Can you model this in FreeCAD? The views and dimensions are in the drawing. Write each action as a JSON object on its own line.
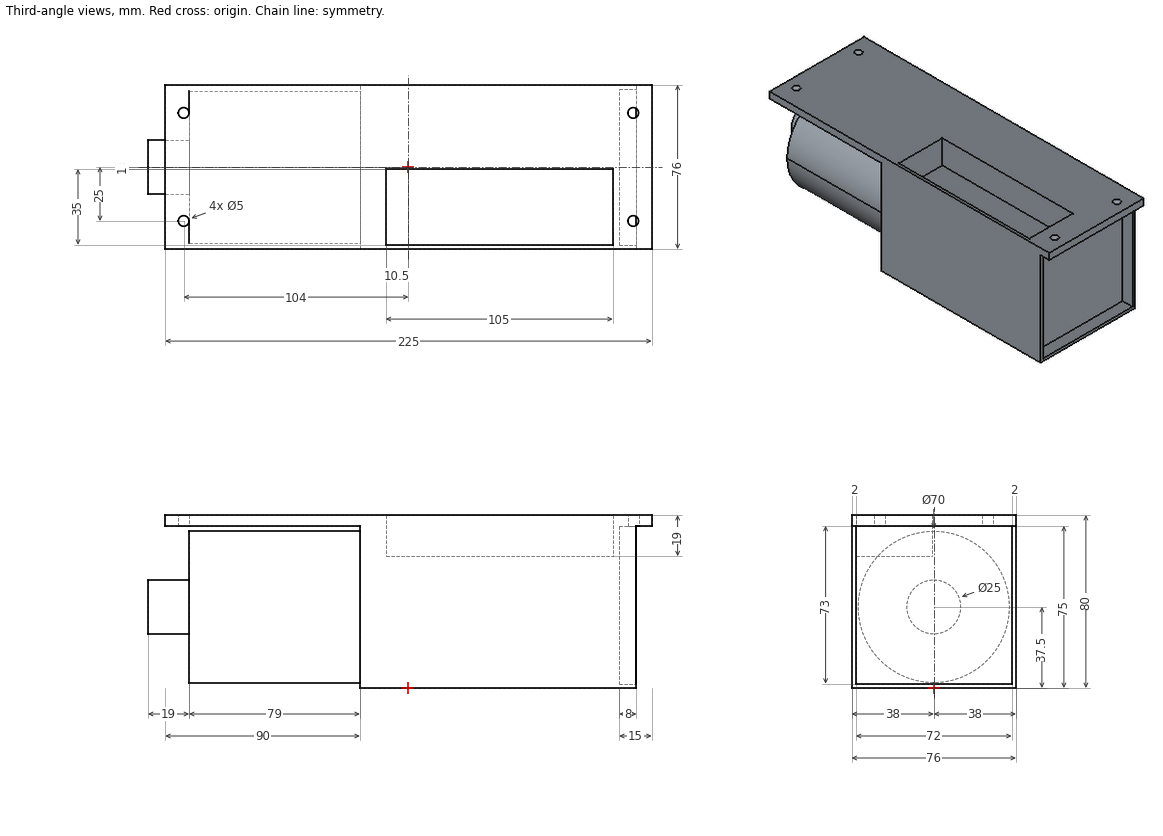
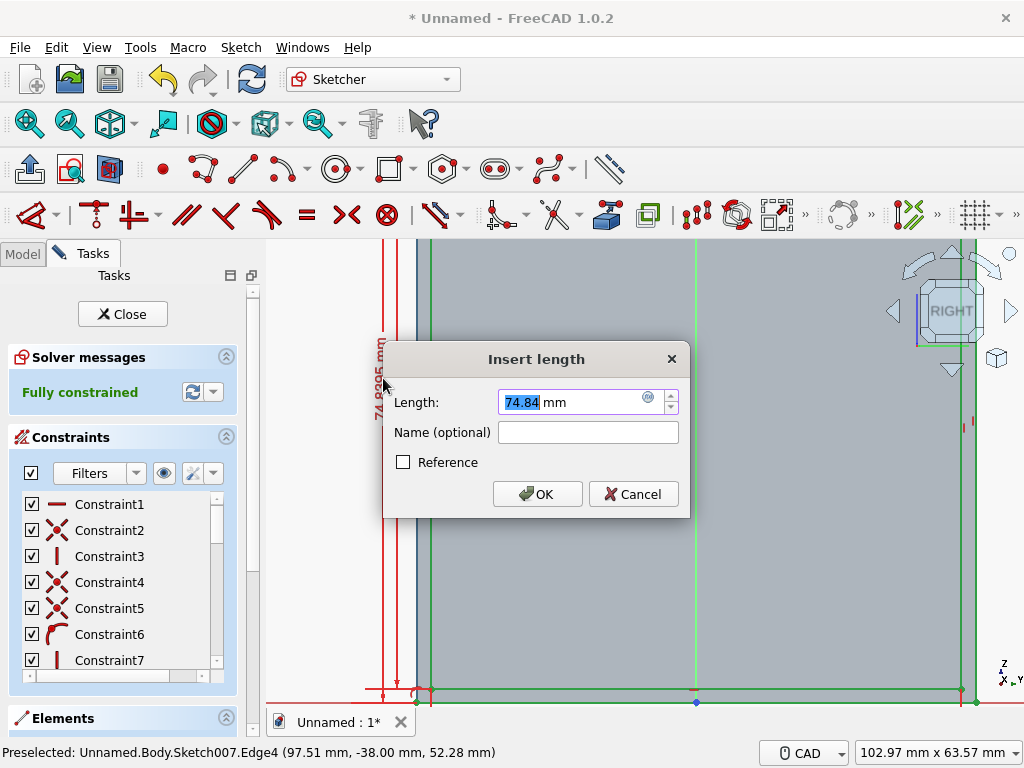
{"action": "type", "text": "75"}
{"action": "key", "text": "Return"}
{"action": "key", "text": "Escape"}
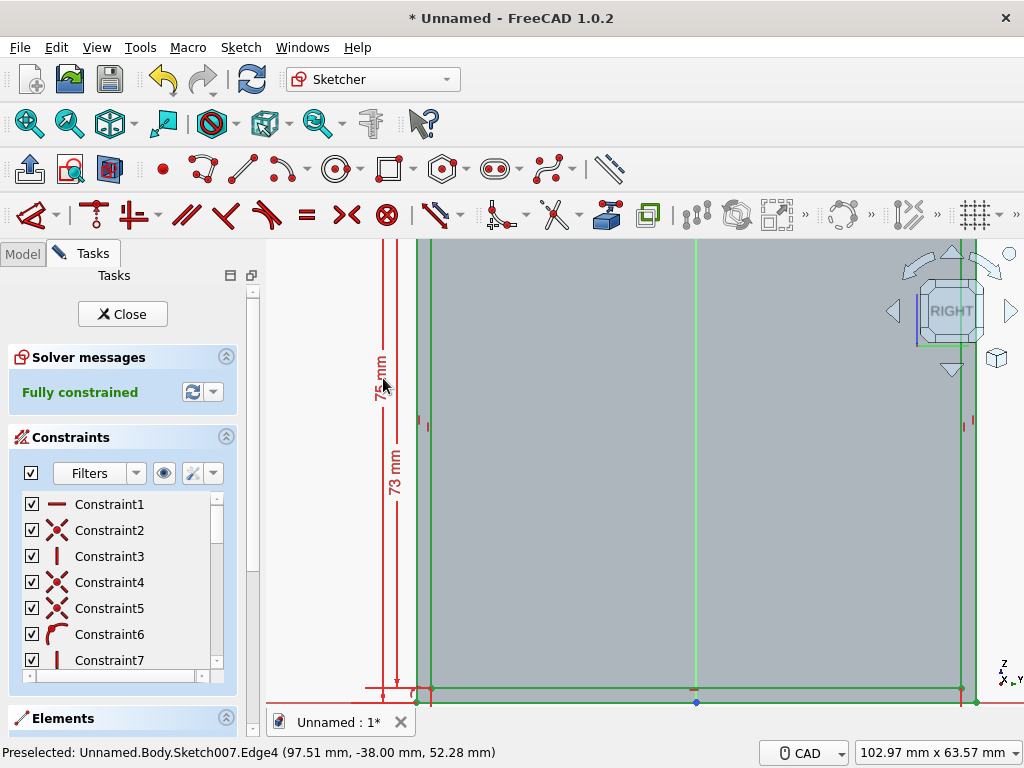
{"action": "left_click", "coordinate": [123, 314]}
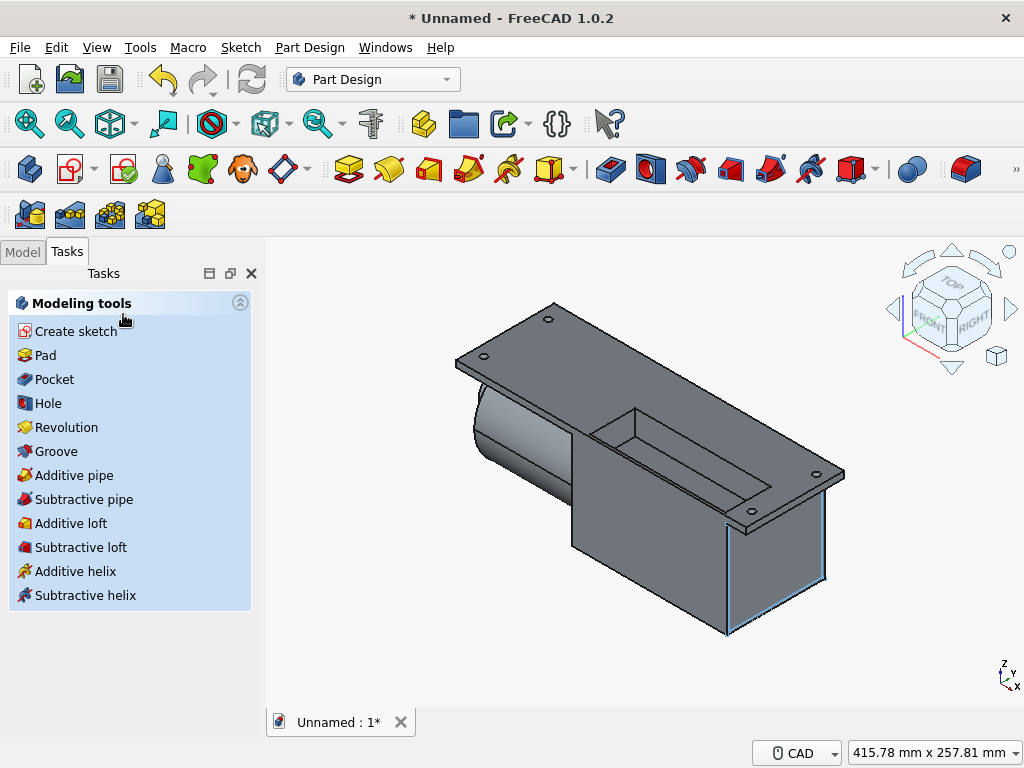
{"action": "left_click", "coordinate": [350, 170]}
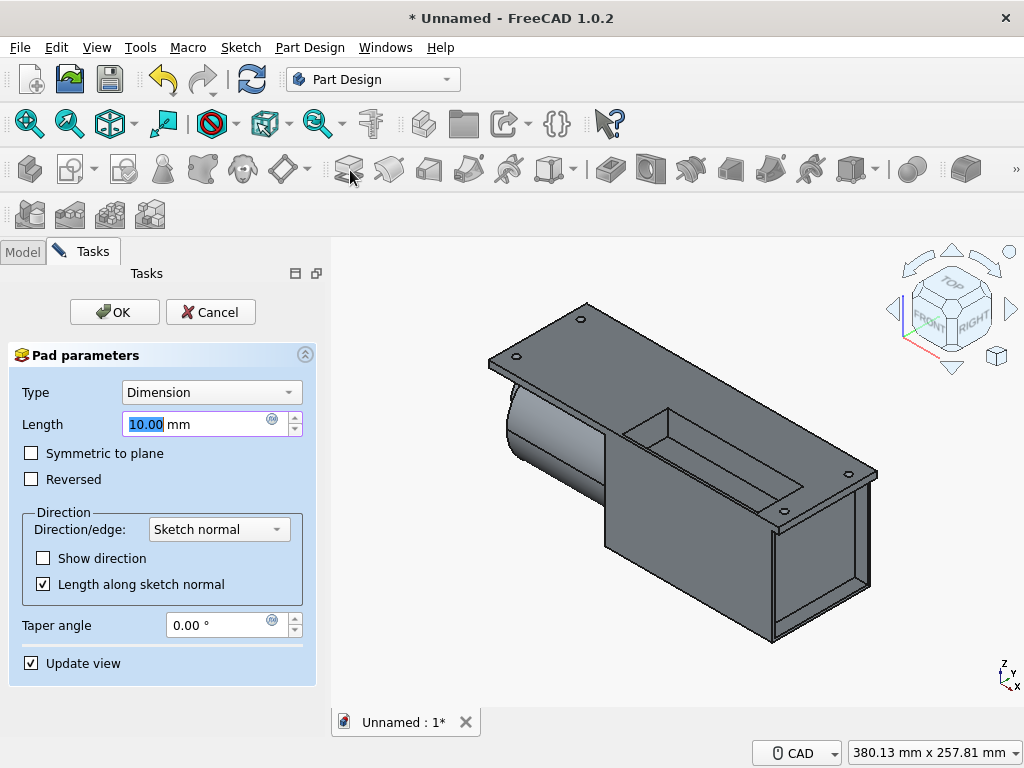
{"action": "type", "text": "8"}
{"action": "key", "text": "Tab"}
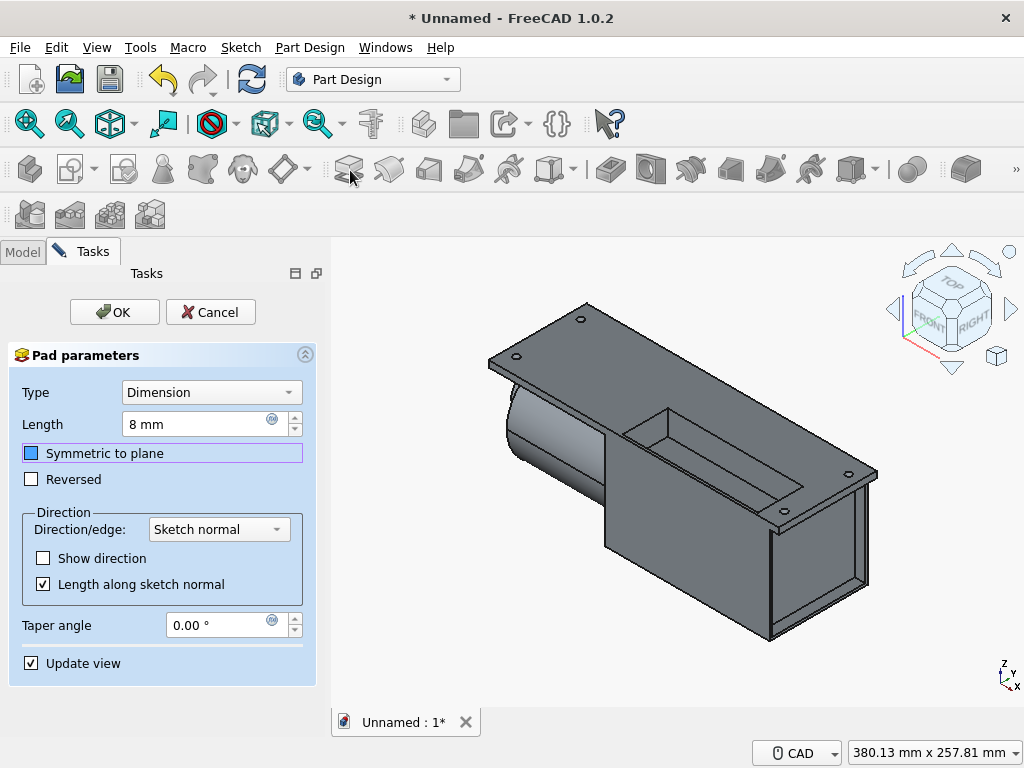
{"action": "left_click", "coordinate": [115, 312]}